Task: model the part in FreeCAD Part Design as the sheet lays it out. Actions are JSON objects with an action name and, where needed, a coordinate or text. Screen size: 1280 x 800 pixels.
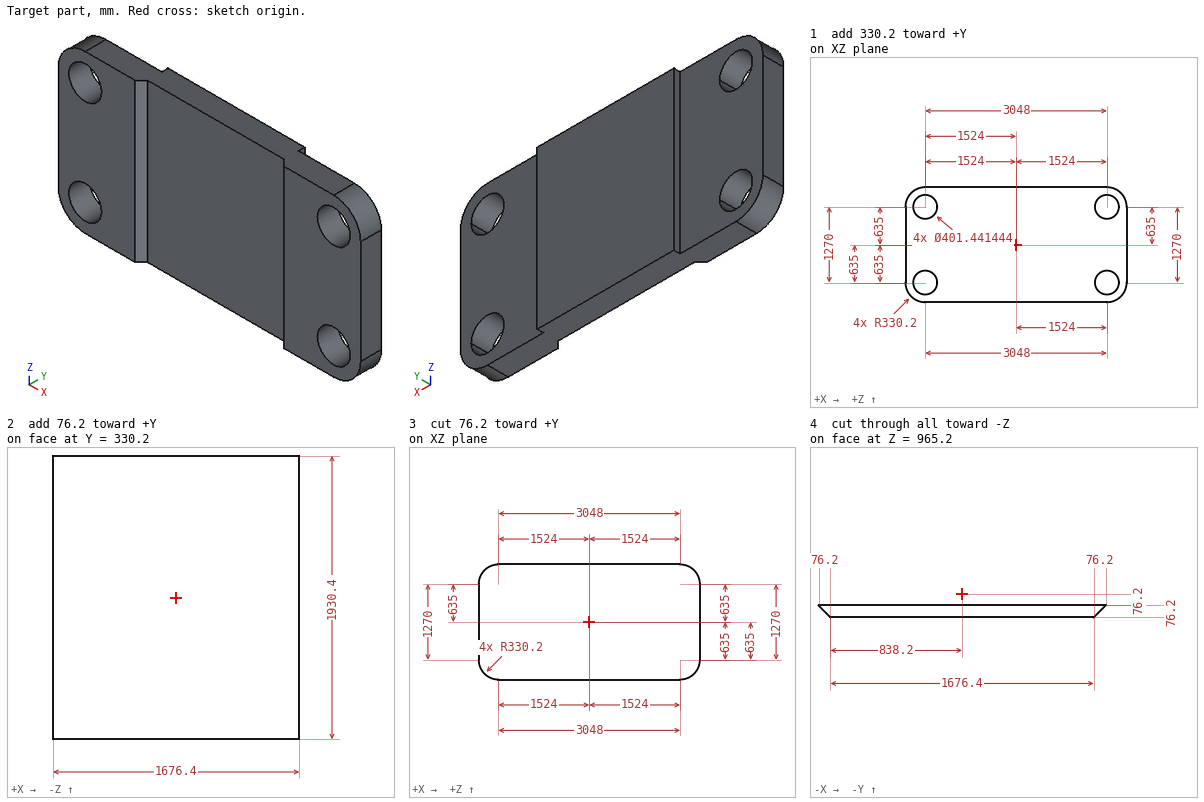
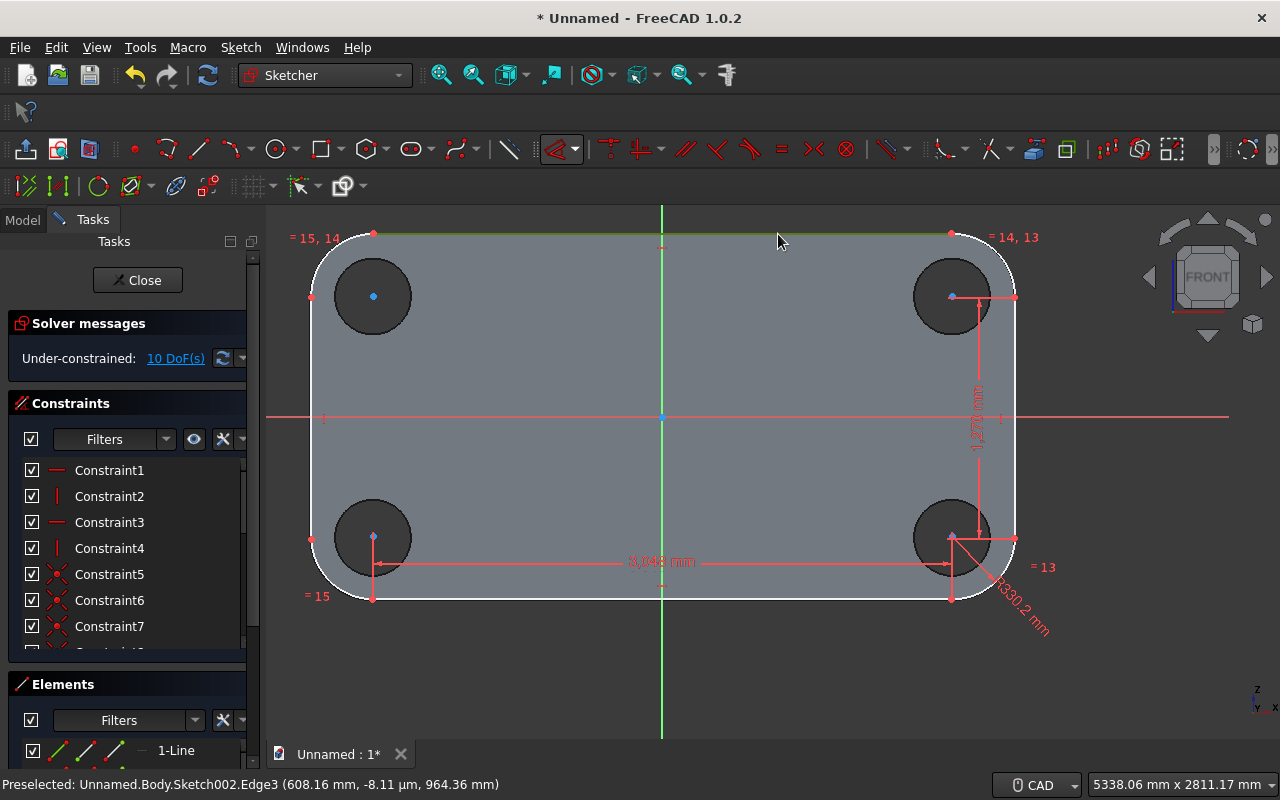
{"action": "key", "text": "l"}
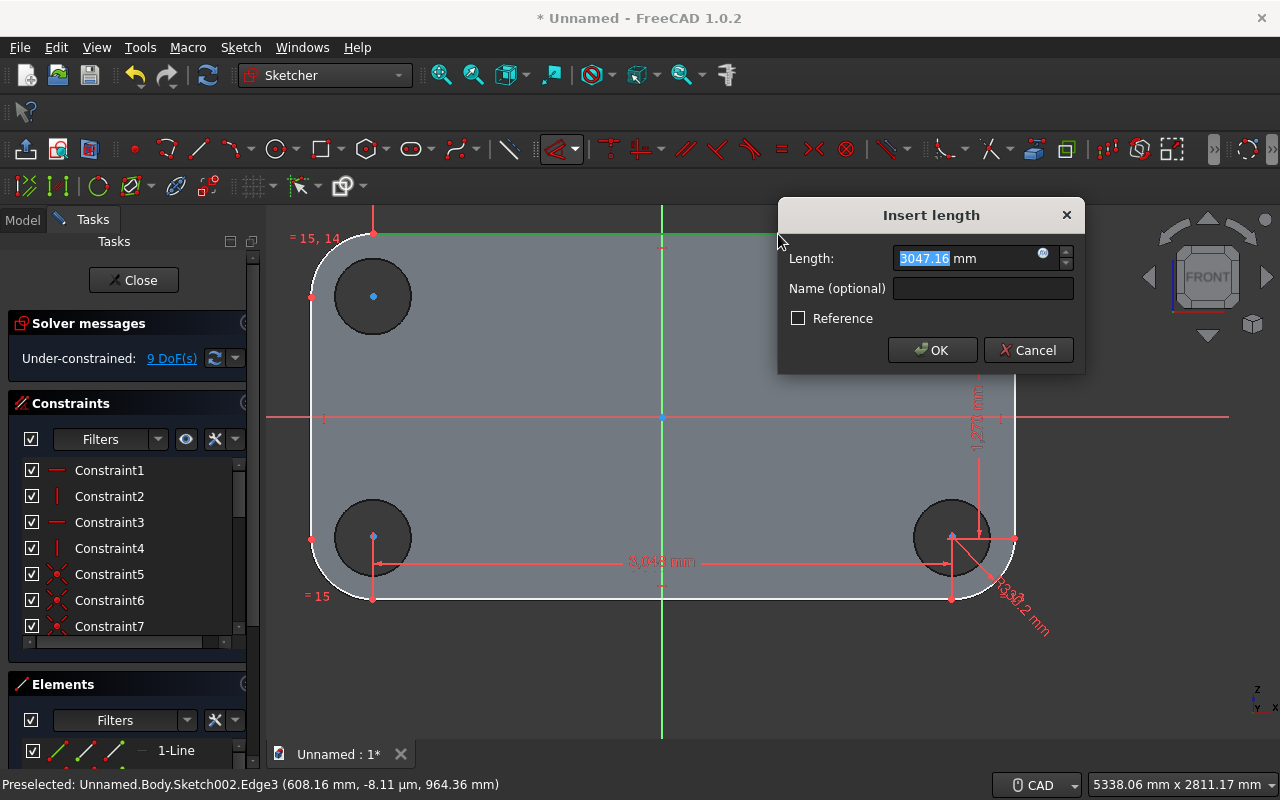
{"action": "type", "text": "3048"}
{"action": "key", "text": "Return"}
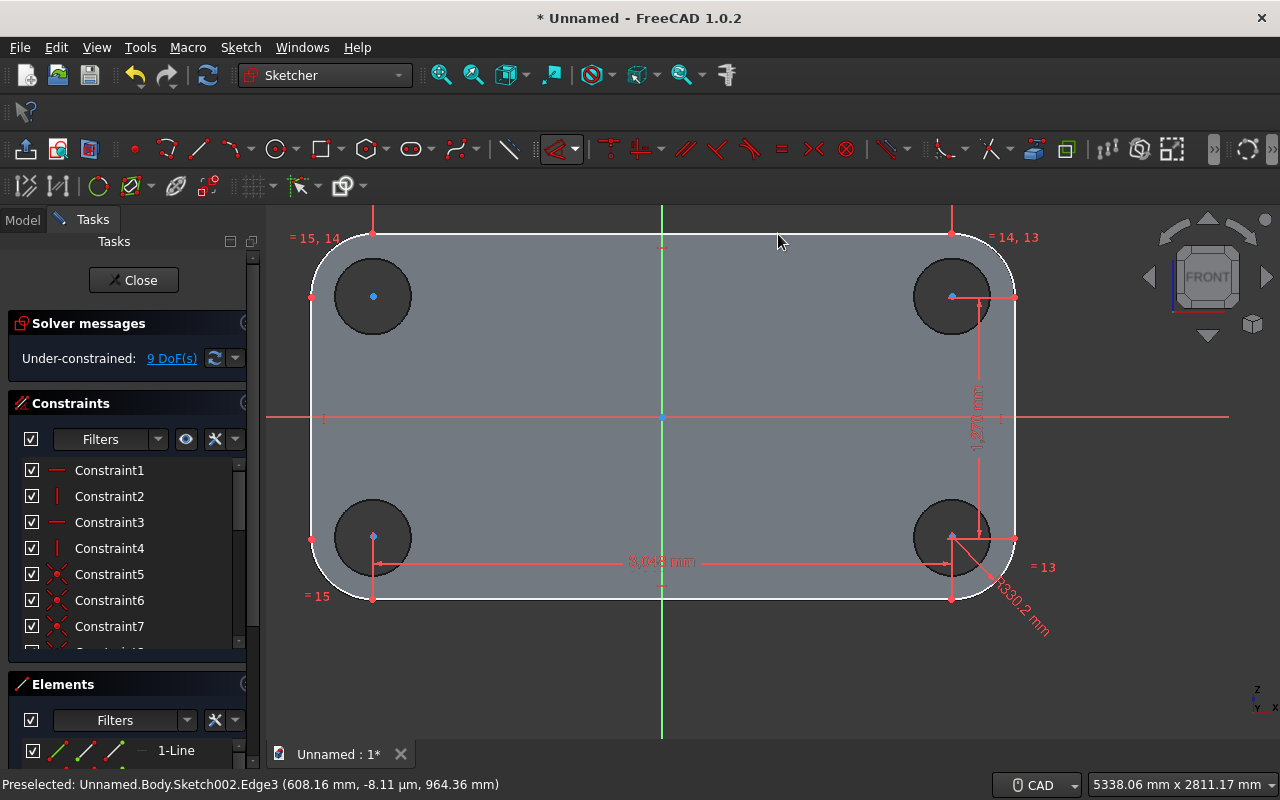
{"action": "left_click", "coordinate": [311, 370]}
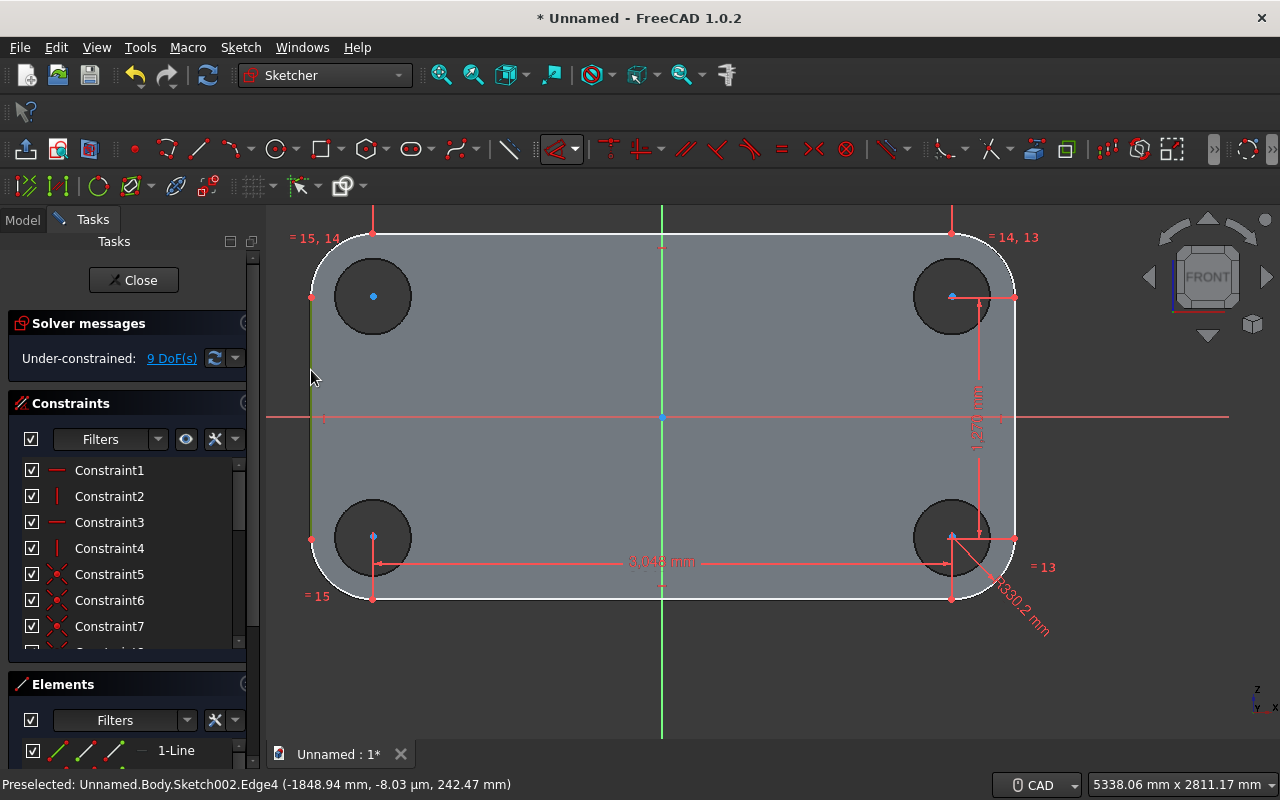
{"action": "key", "text": "i"}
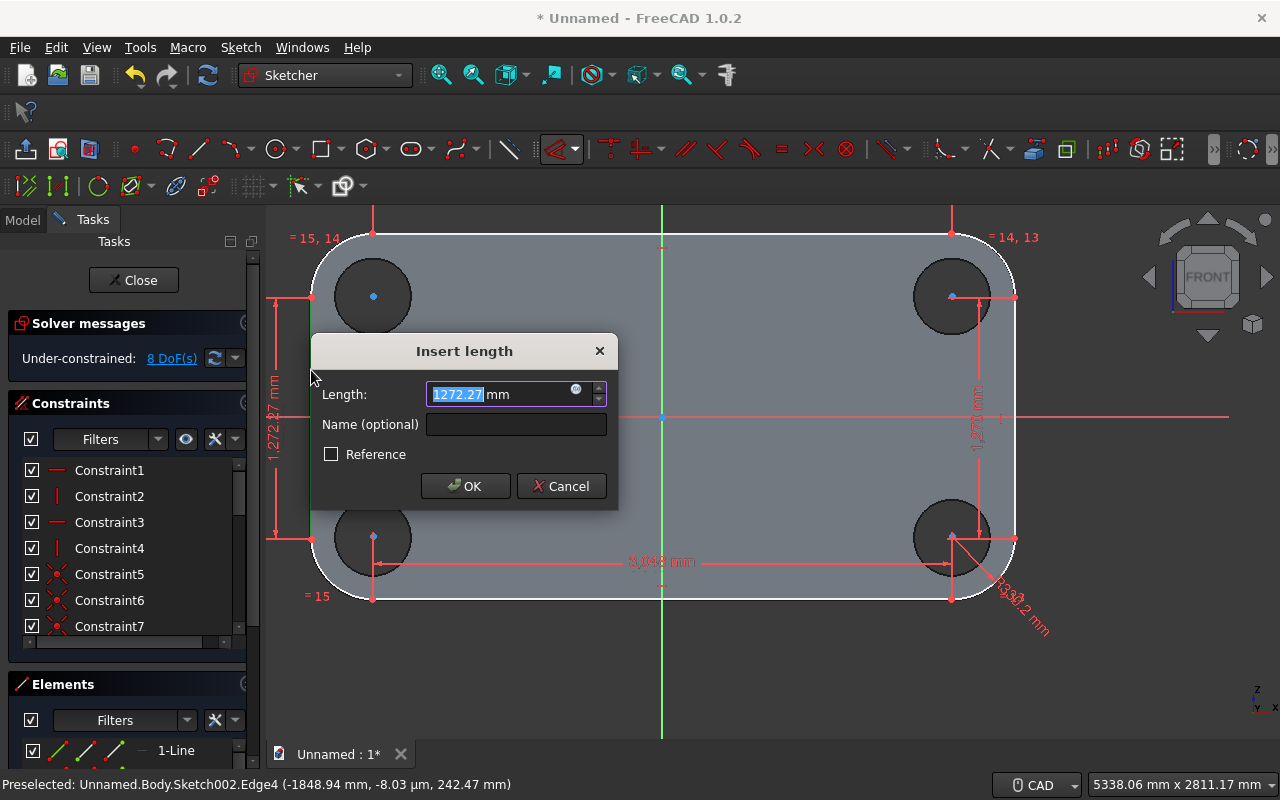
{"action": "type", "text": "1270"}
{"action": "key", "text": "Return"}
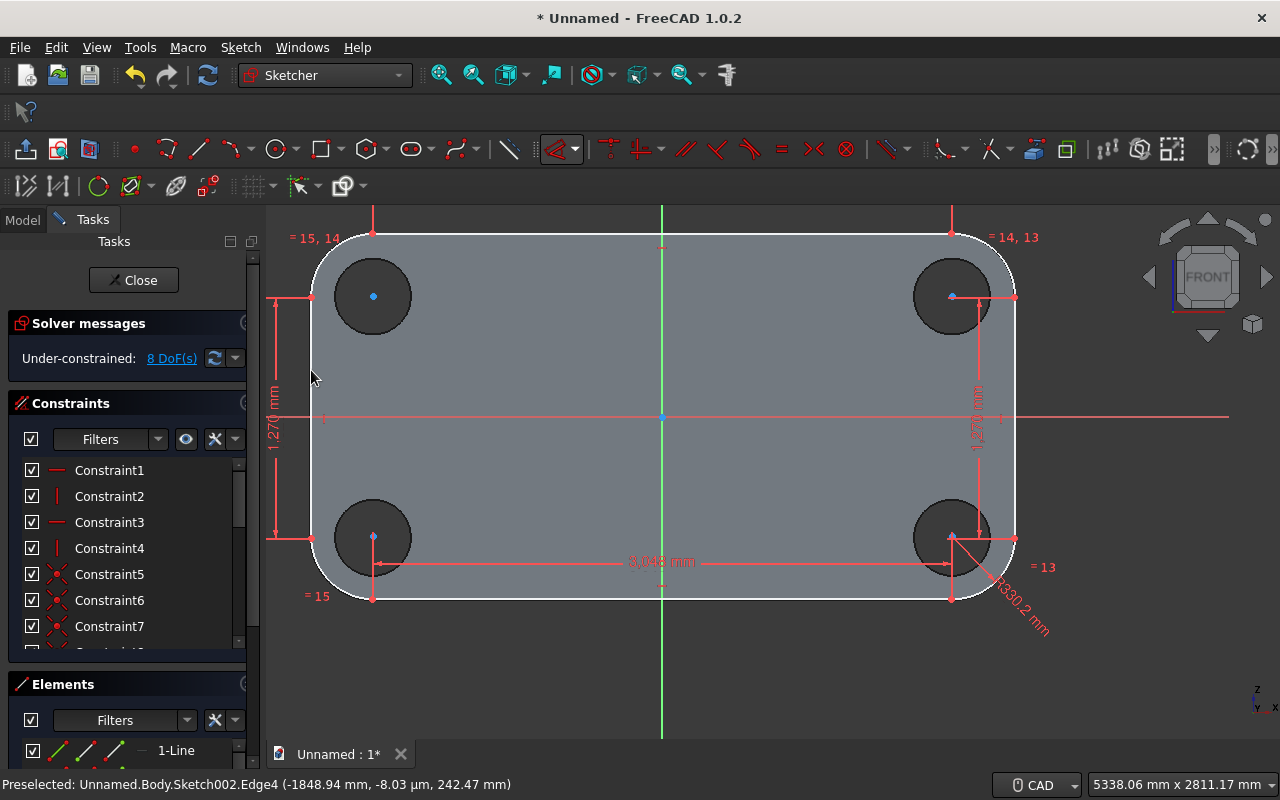
{"action": "left_click", "coordinate": [1015, 539]}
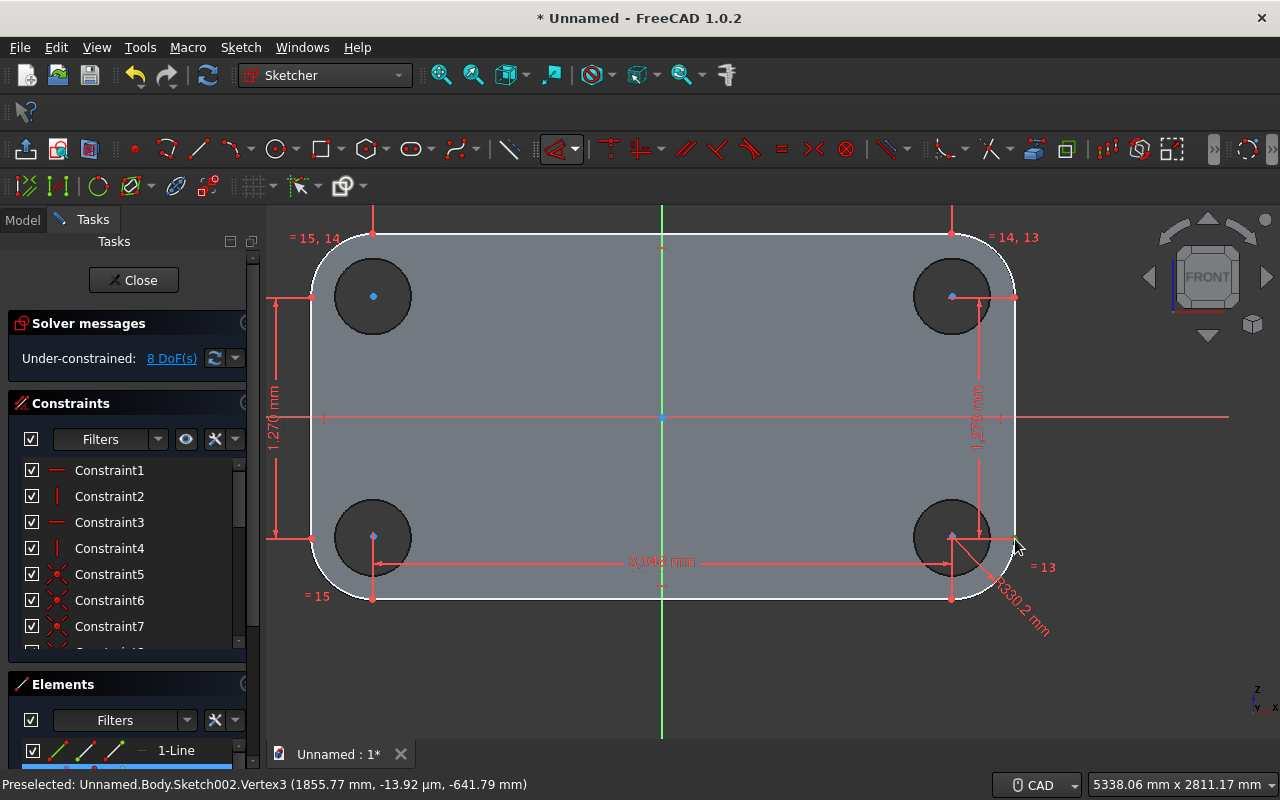
{"action": "key", "text": "i"}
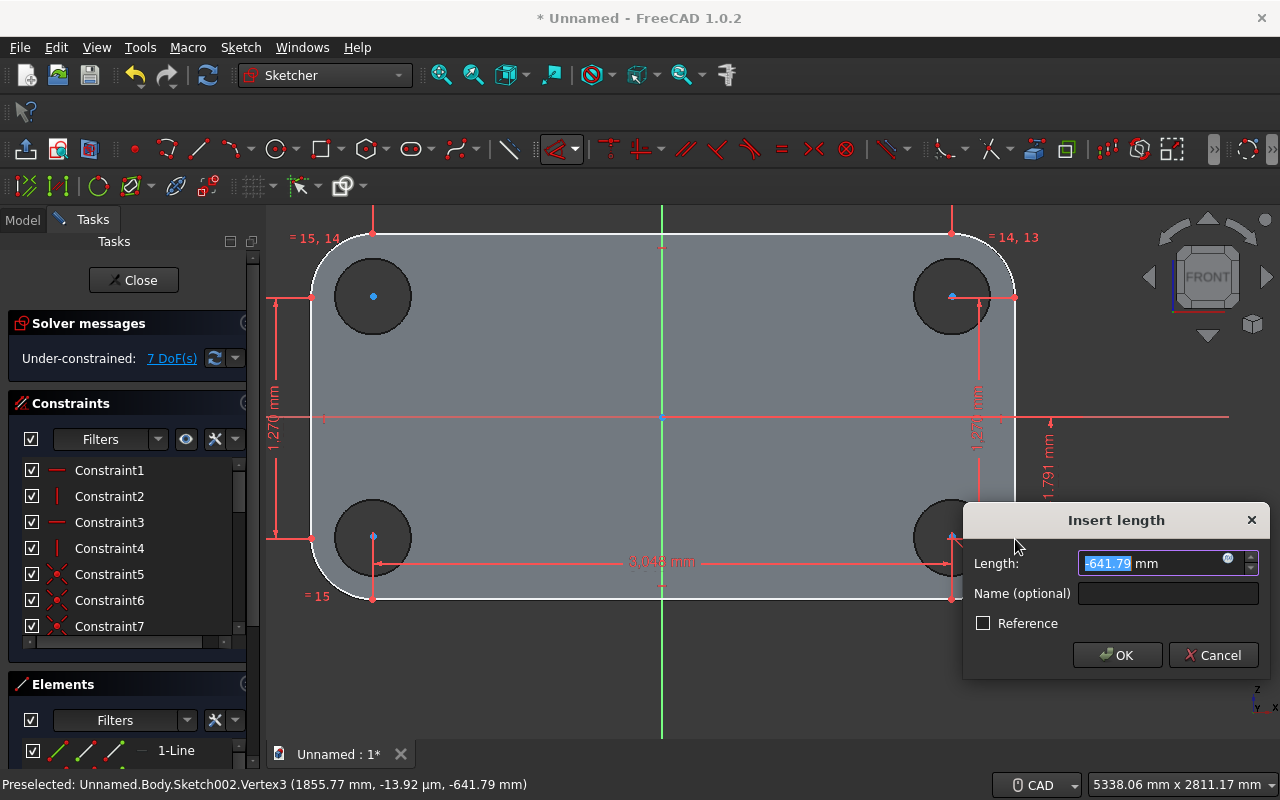
{"action": "type", "text": "-635"}
{"action": "key", "text": "Return"}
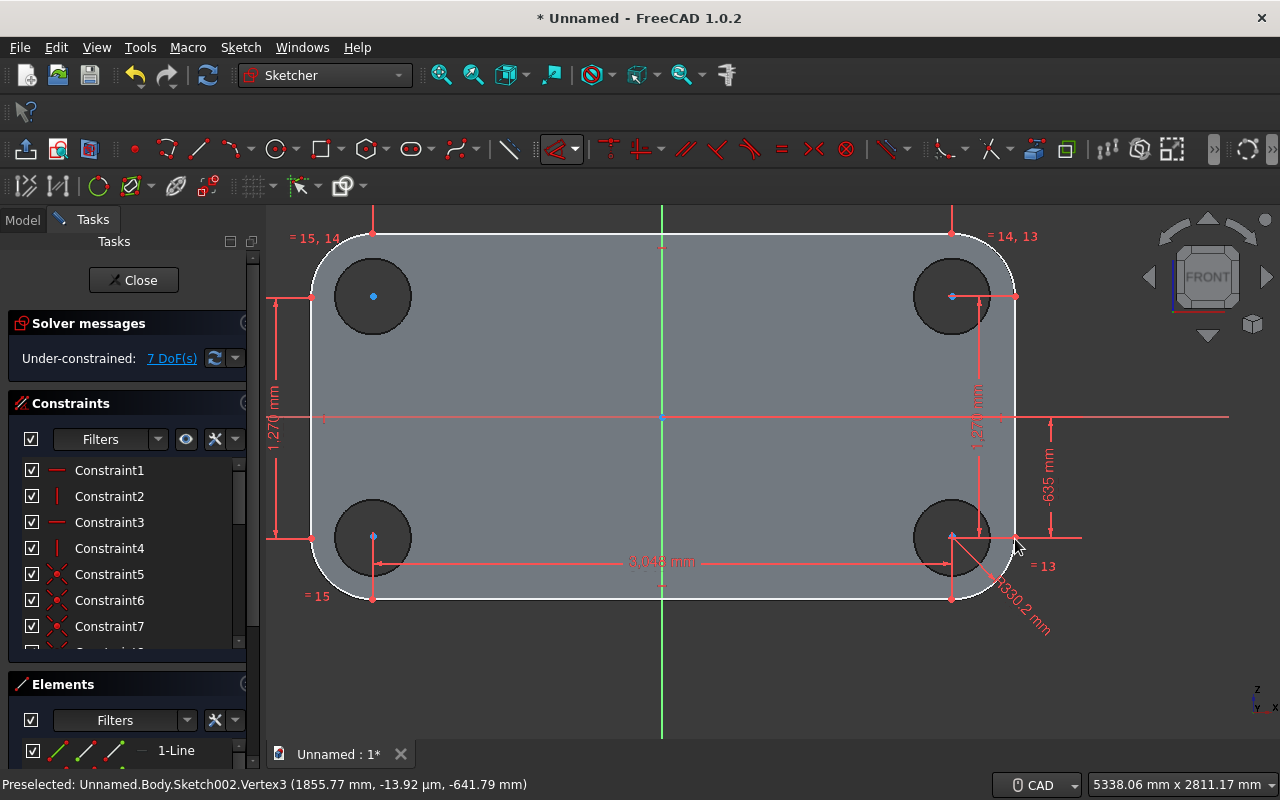
{"action": "left_click", "coordinate": [311, 298]}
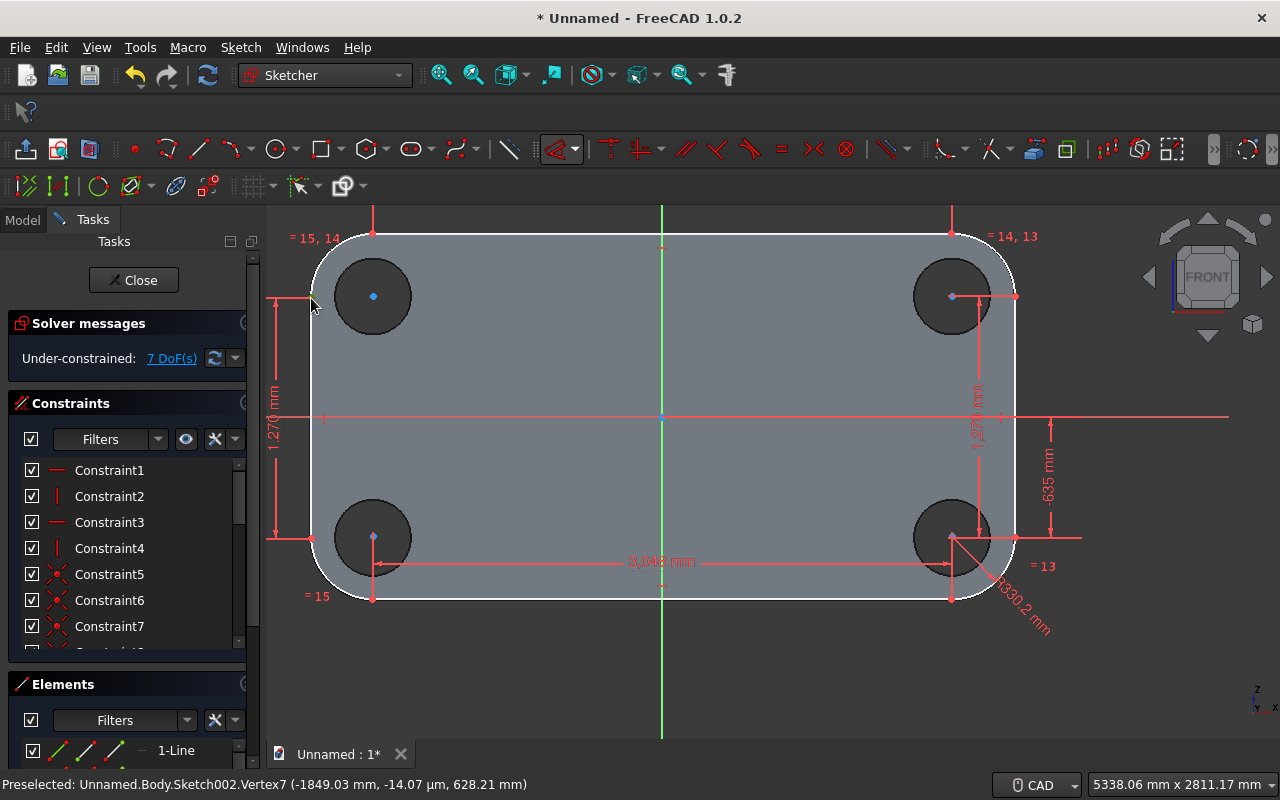
{"action": "key", "text": "i"}